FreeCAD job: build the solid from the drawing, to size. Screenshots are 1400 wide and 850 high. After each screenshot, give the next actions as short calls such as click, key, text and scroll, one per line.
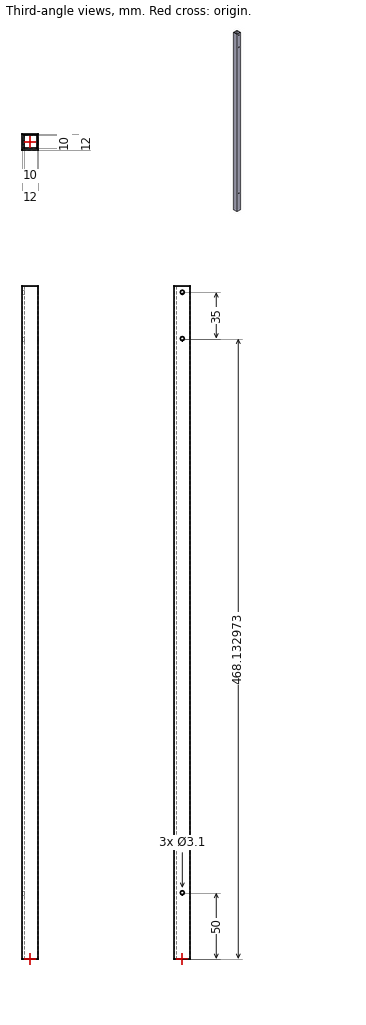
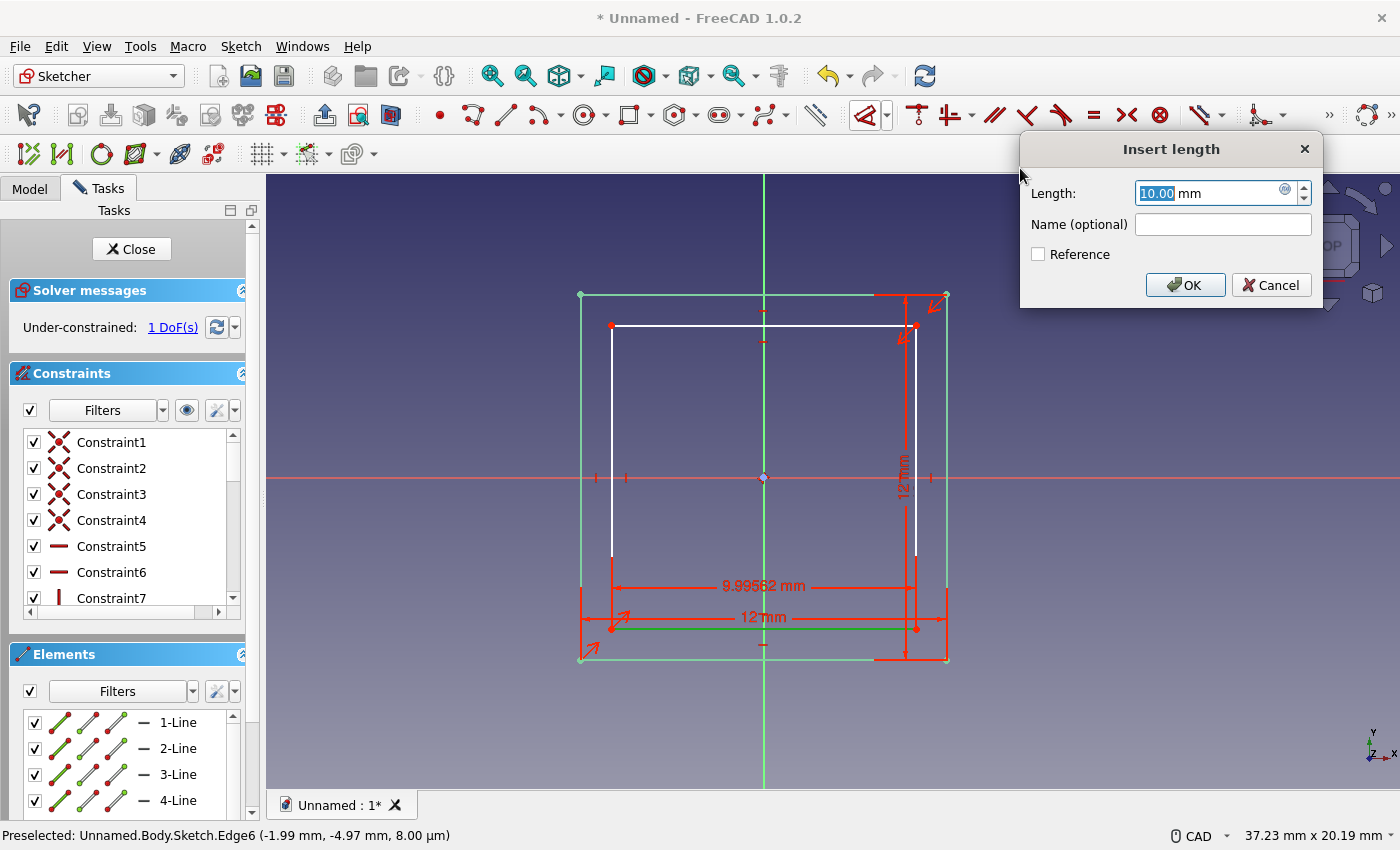
text(10)
key(Return)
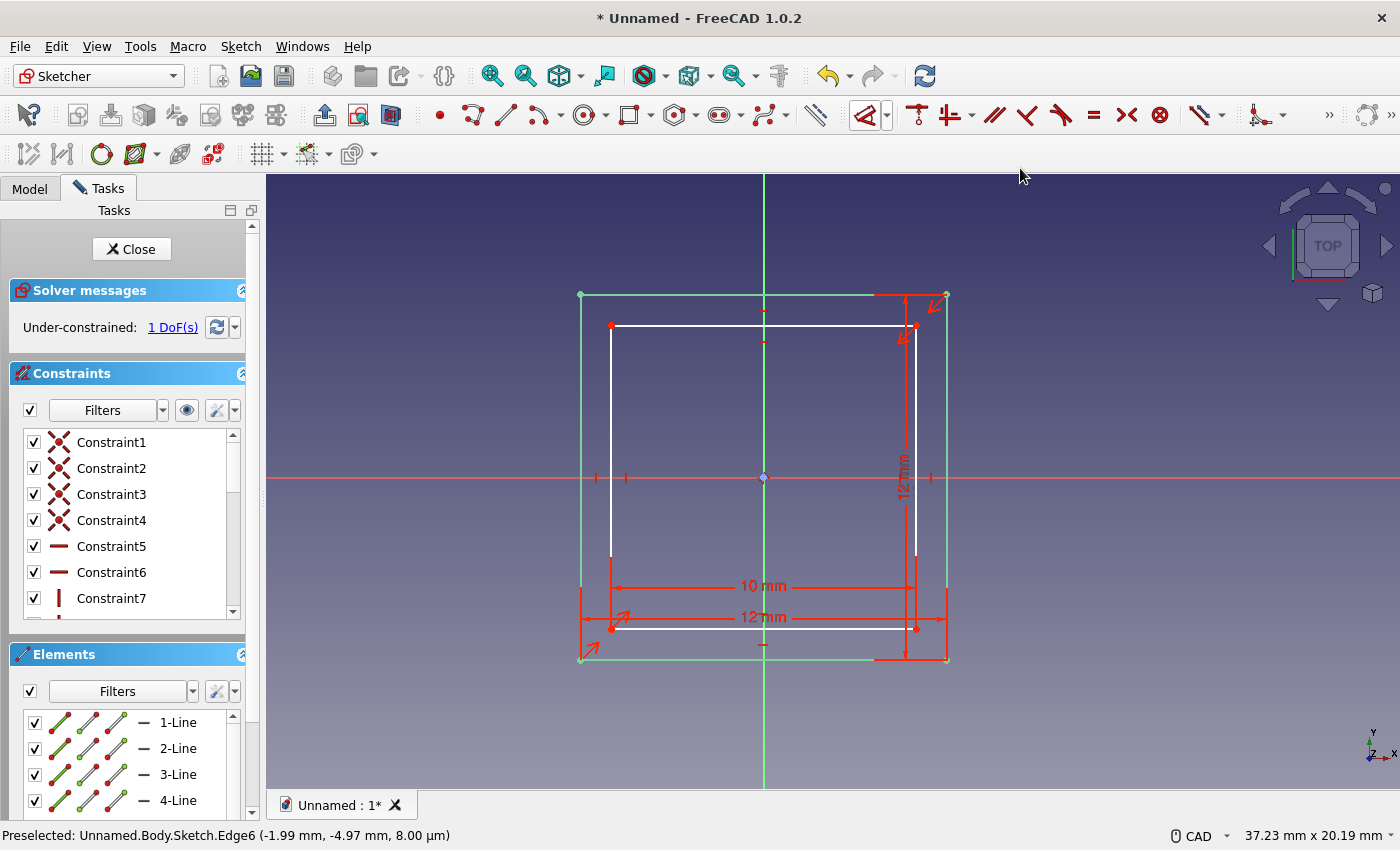
click(916, 538)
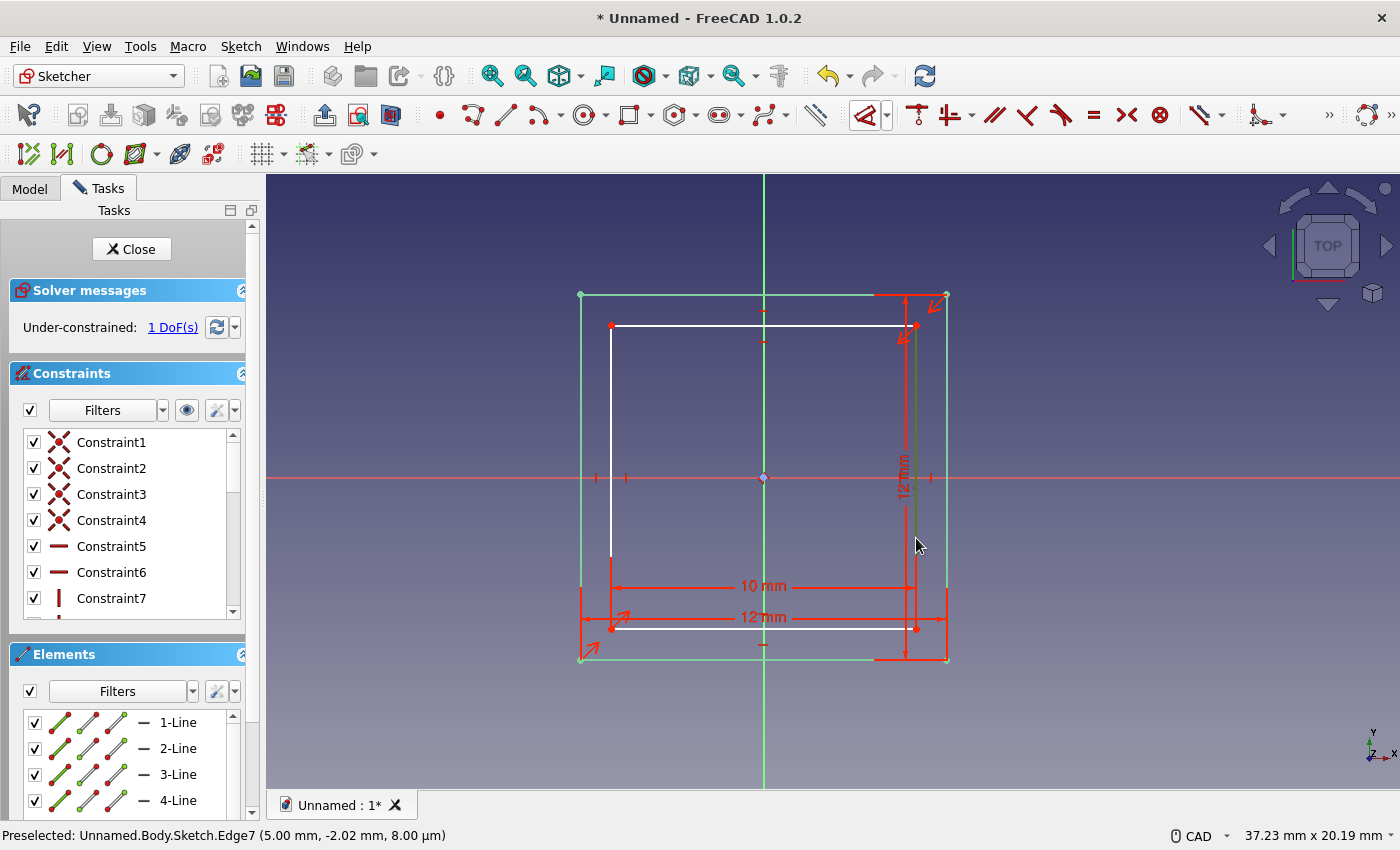
key(i)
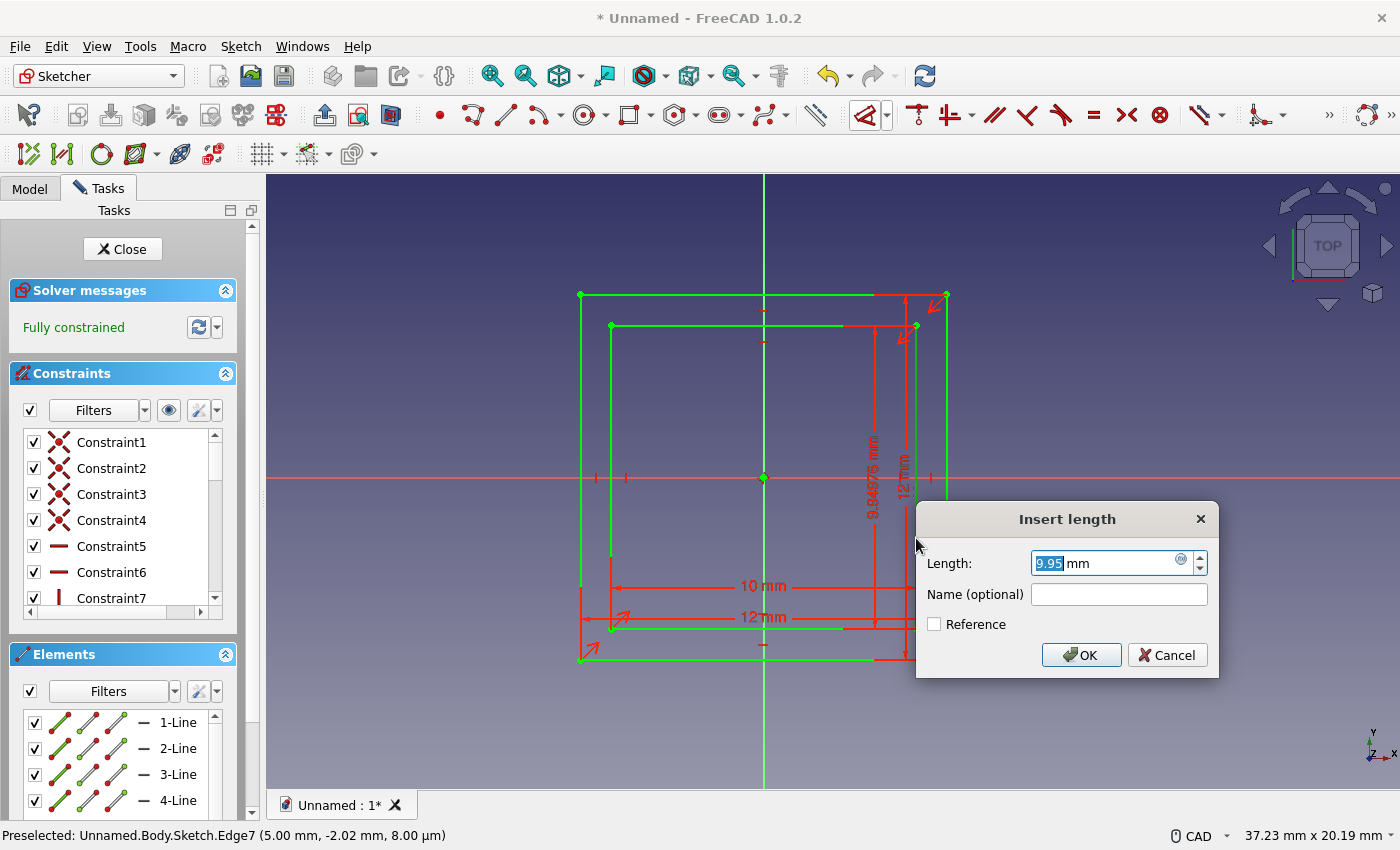
text(10)
key(Return)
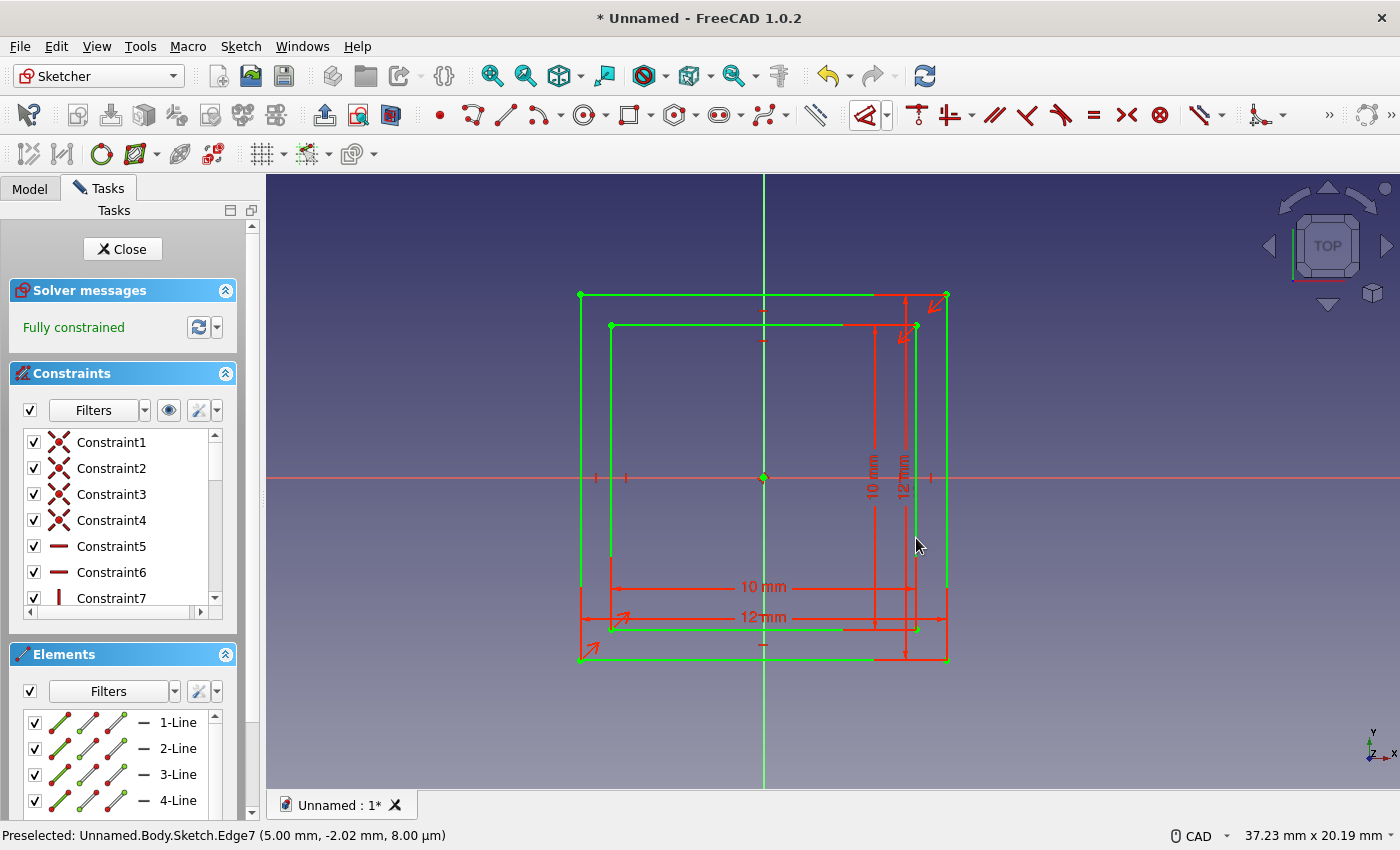
click(123, 249)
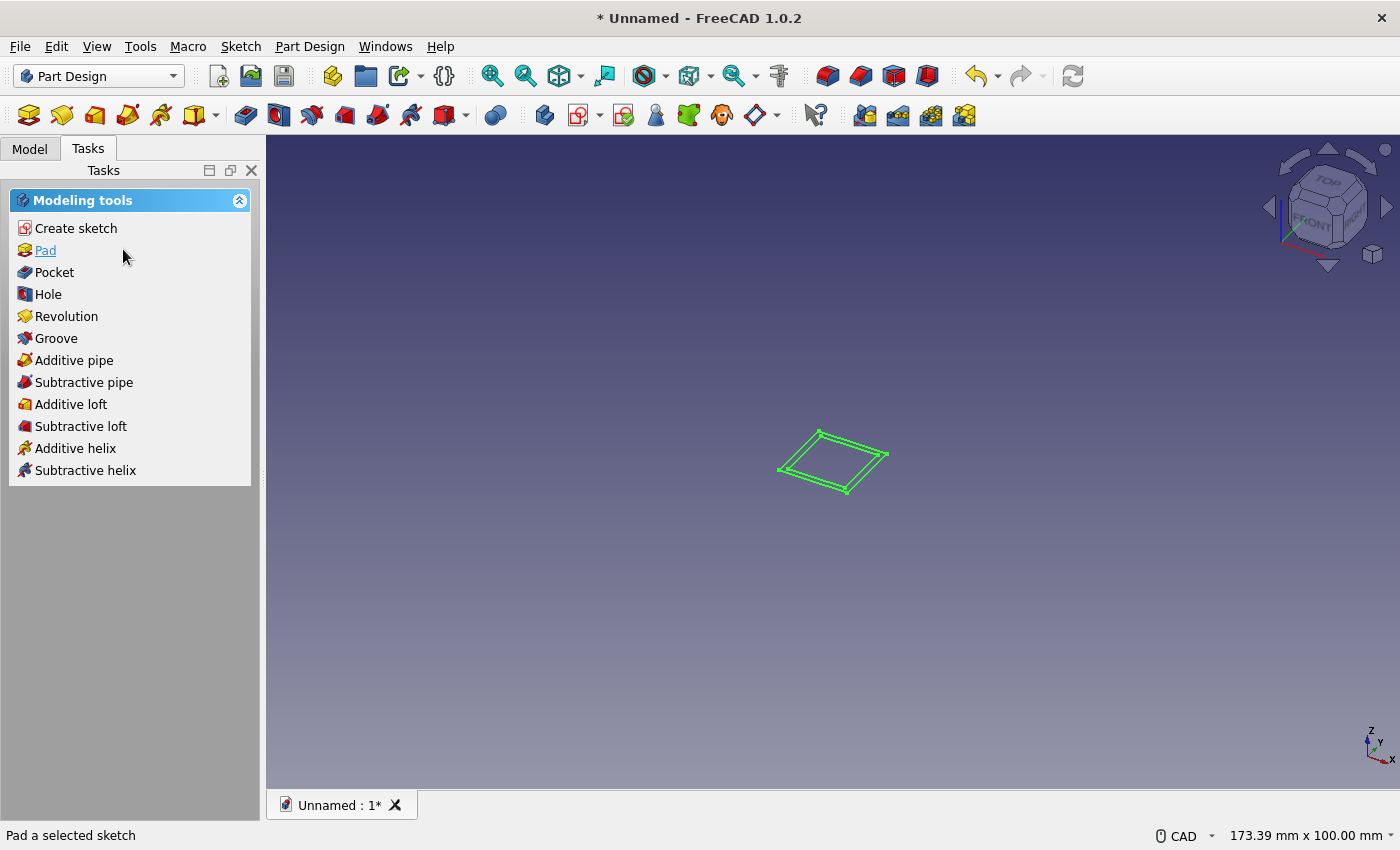
click(29, 116)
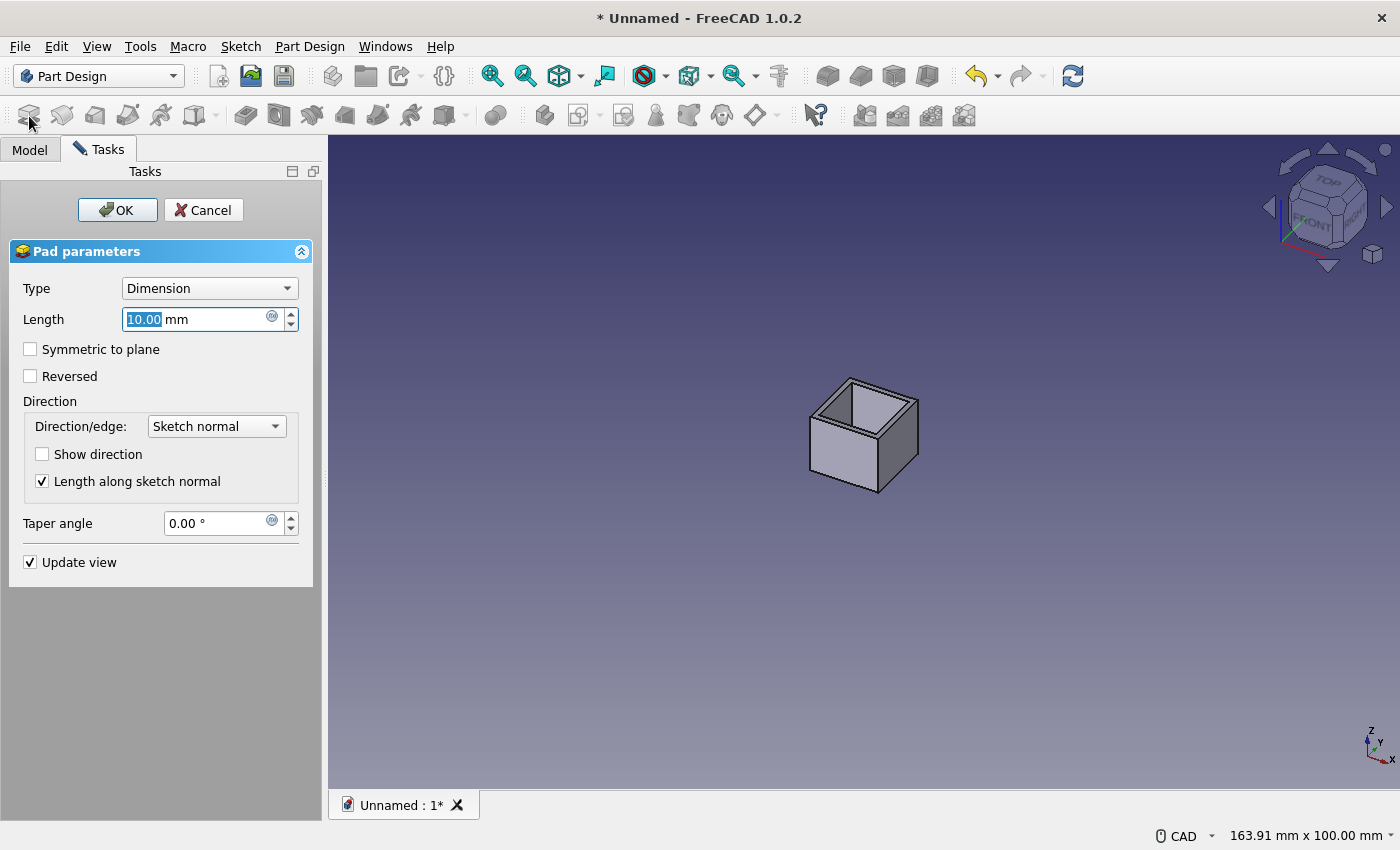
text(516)
key(Tab)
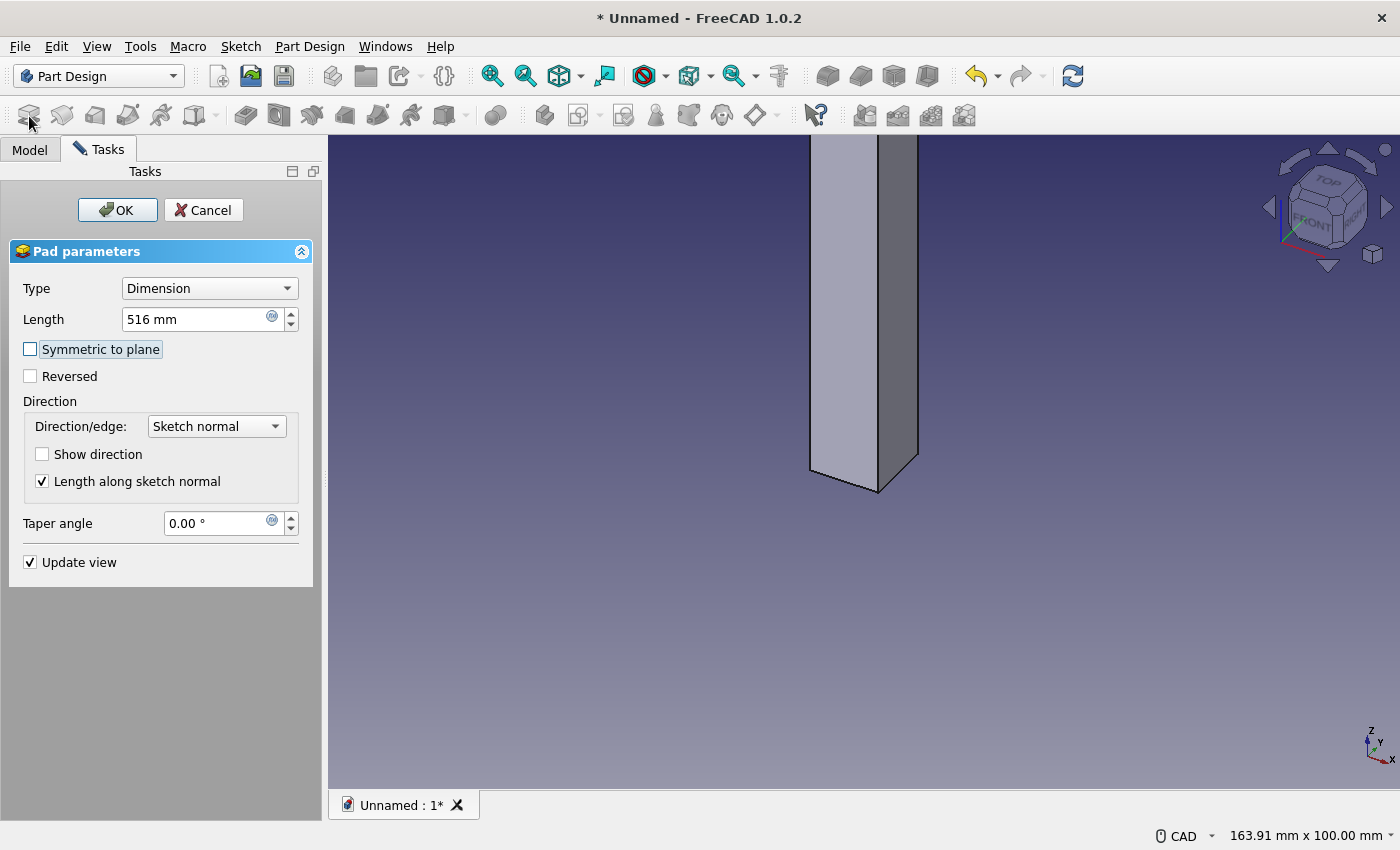
click(118, 210)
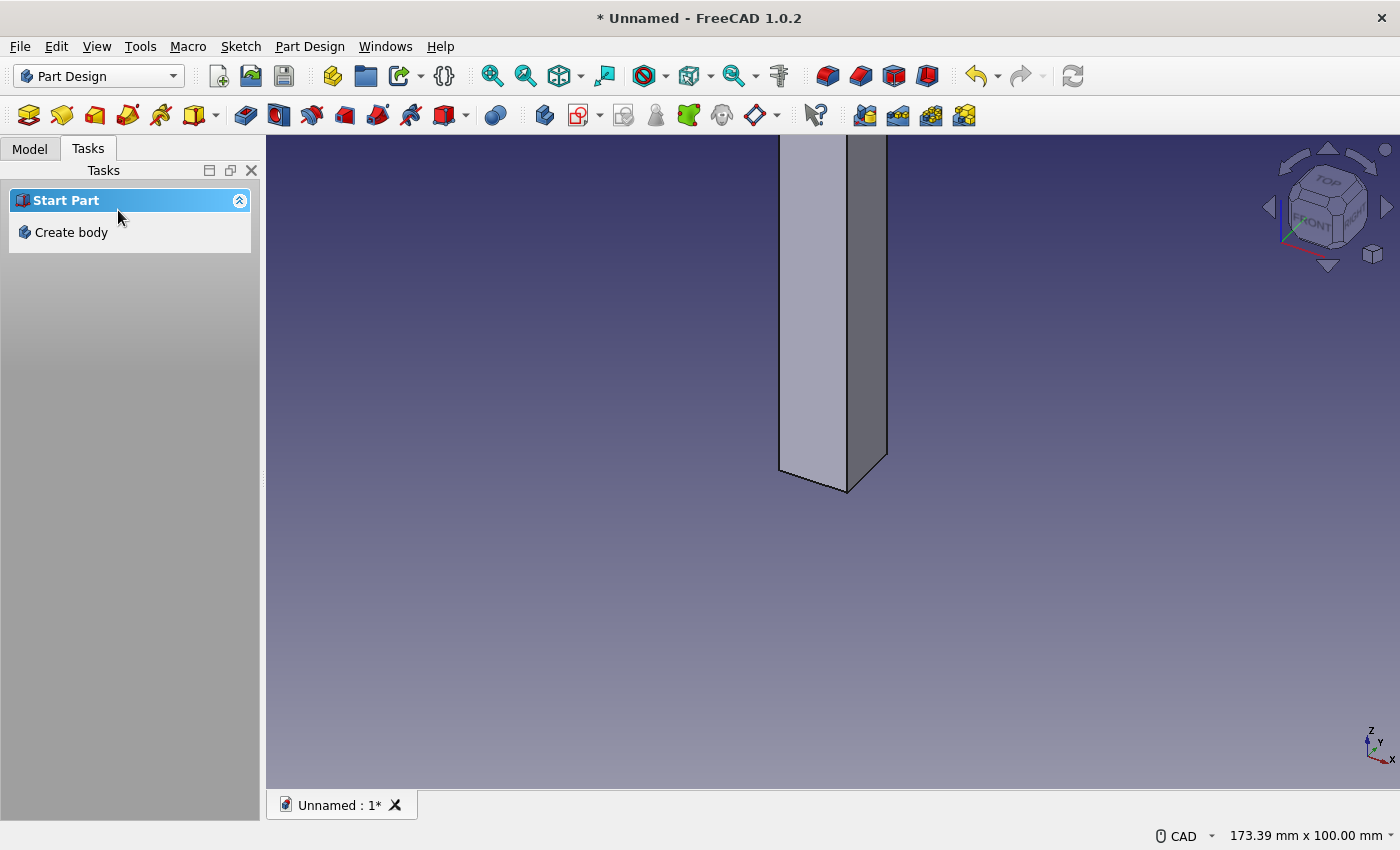
click(493, 76)